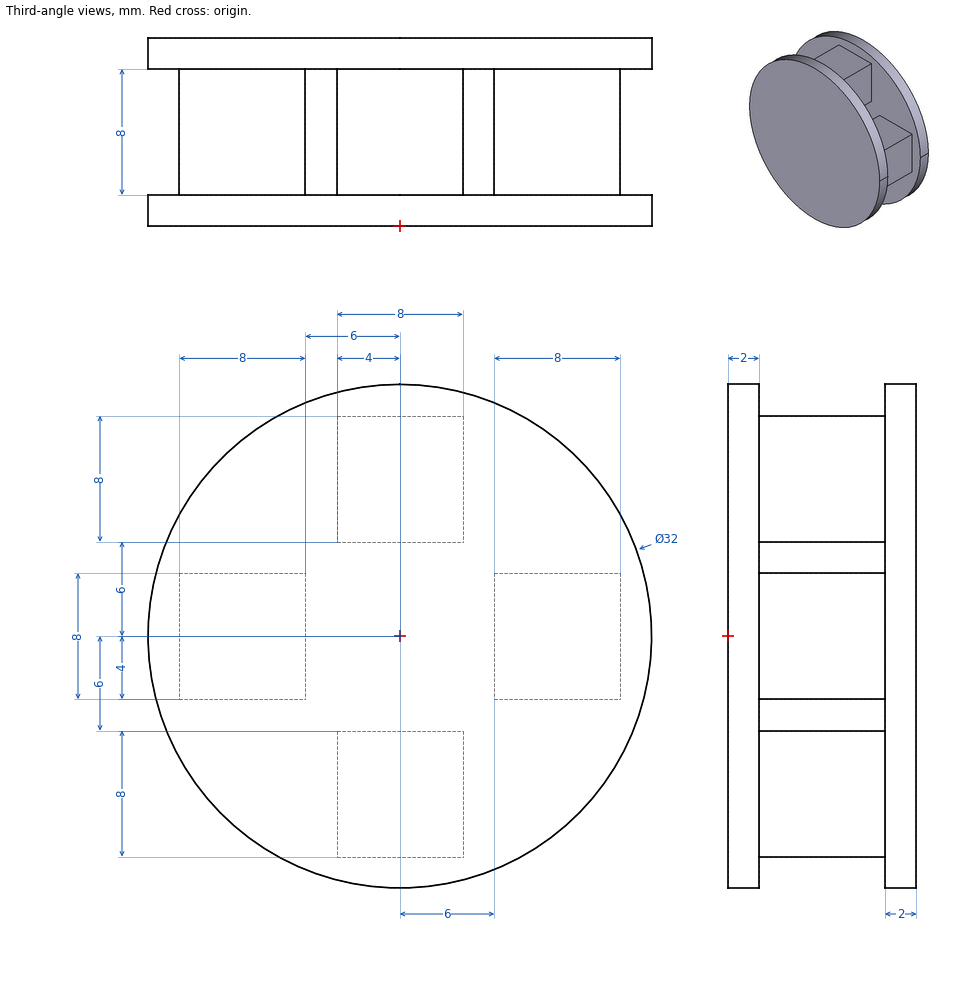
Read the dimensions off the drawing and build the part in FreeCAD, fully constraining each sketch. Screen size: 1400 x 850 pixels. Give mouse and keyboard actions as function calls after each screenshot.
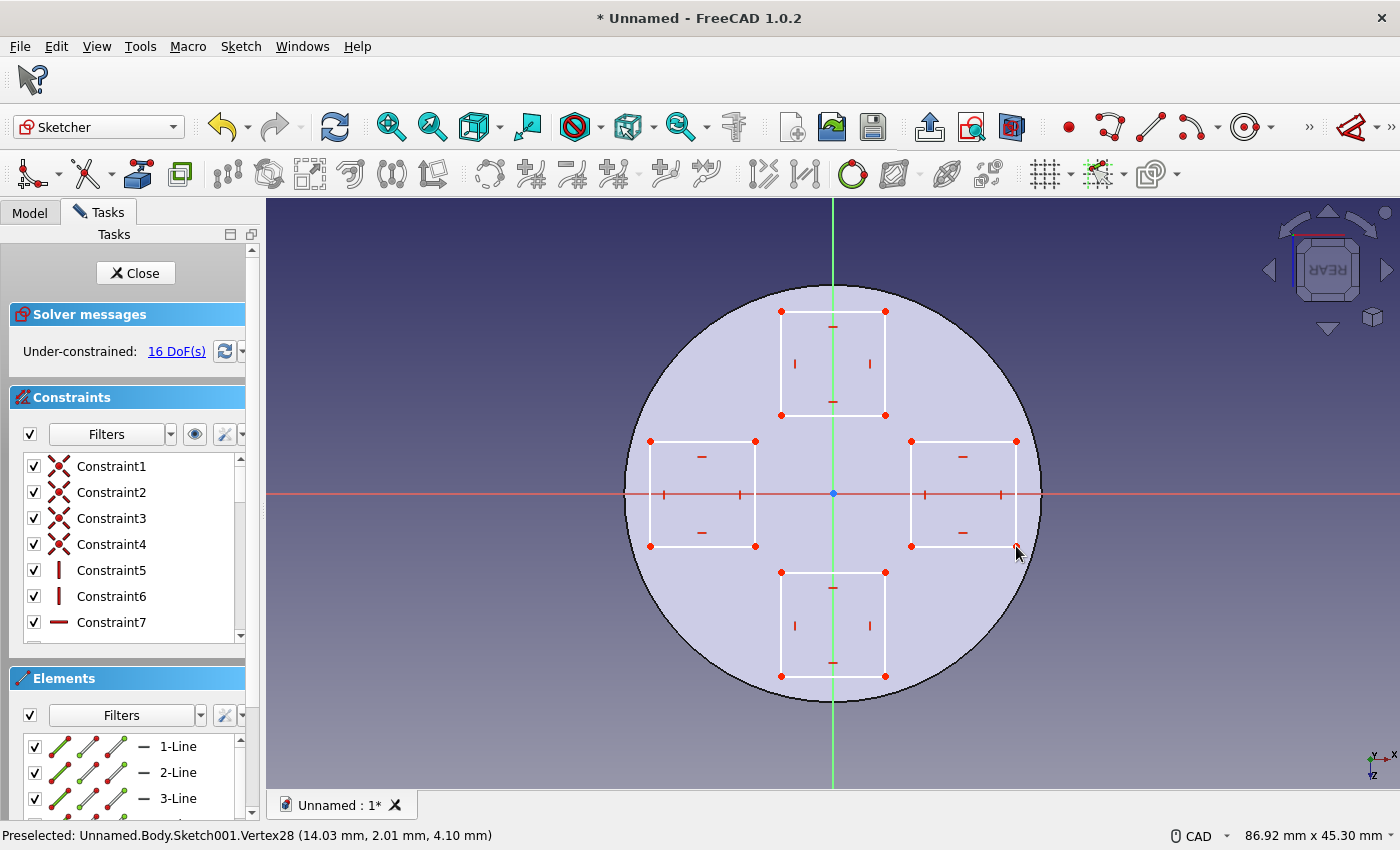
key(d)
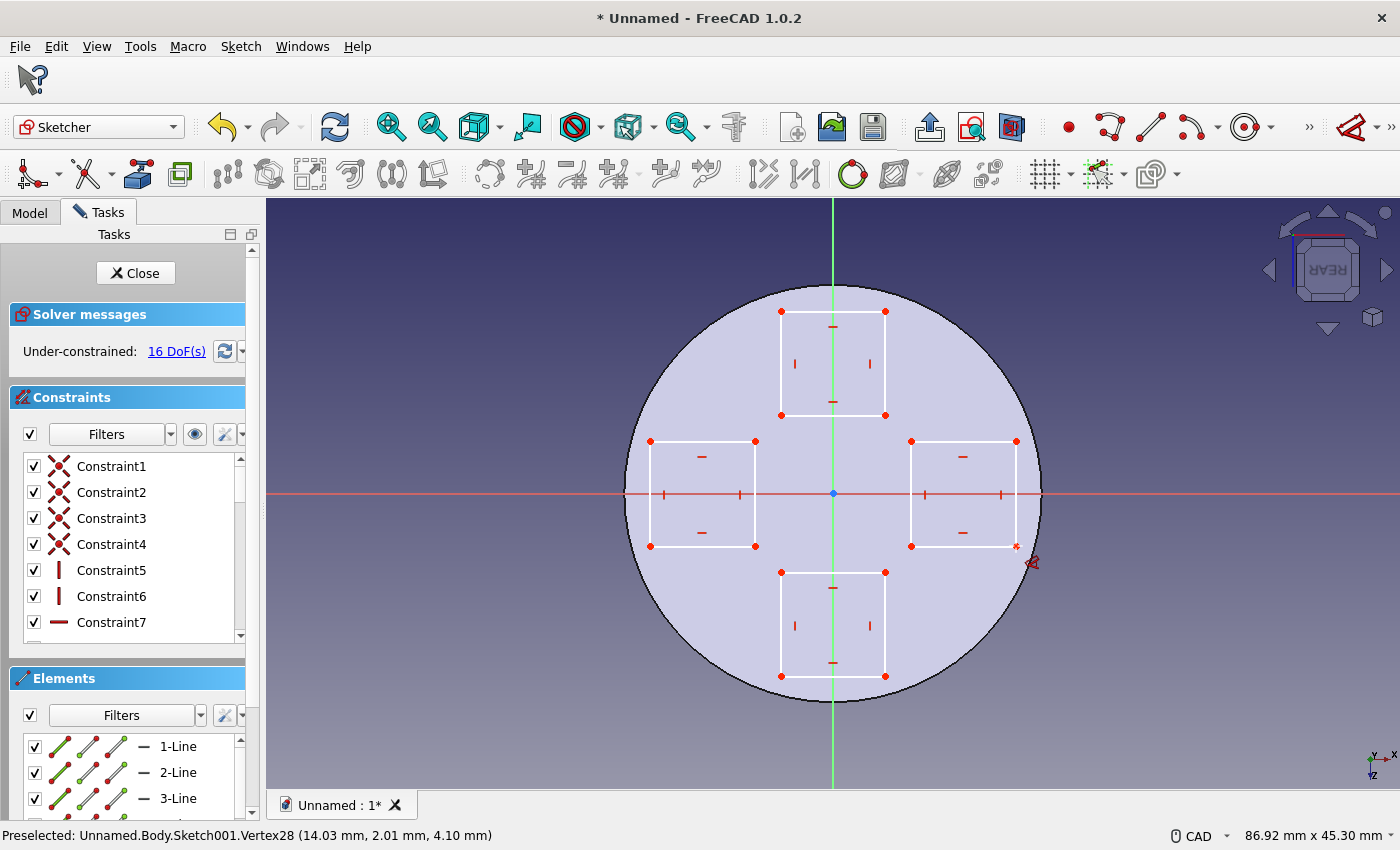
click(650, 473)
click(616, 470)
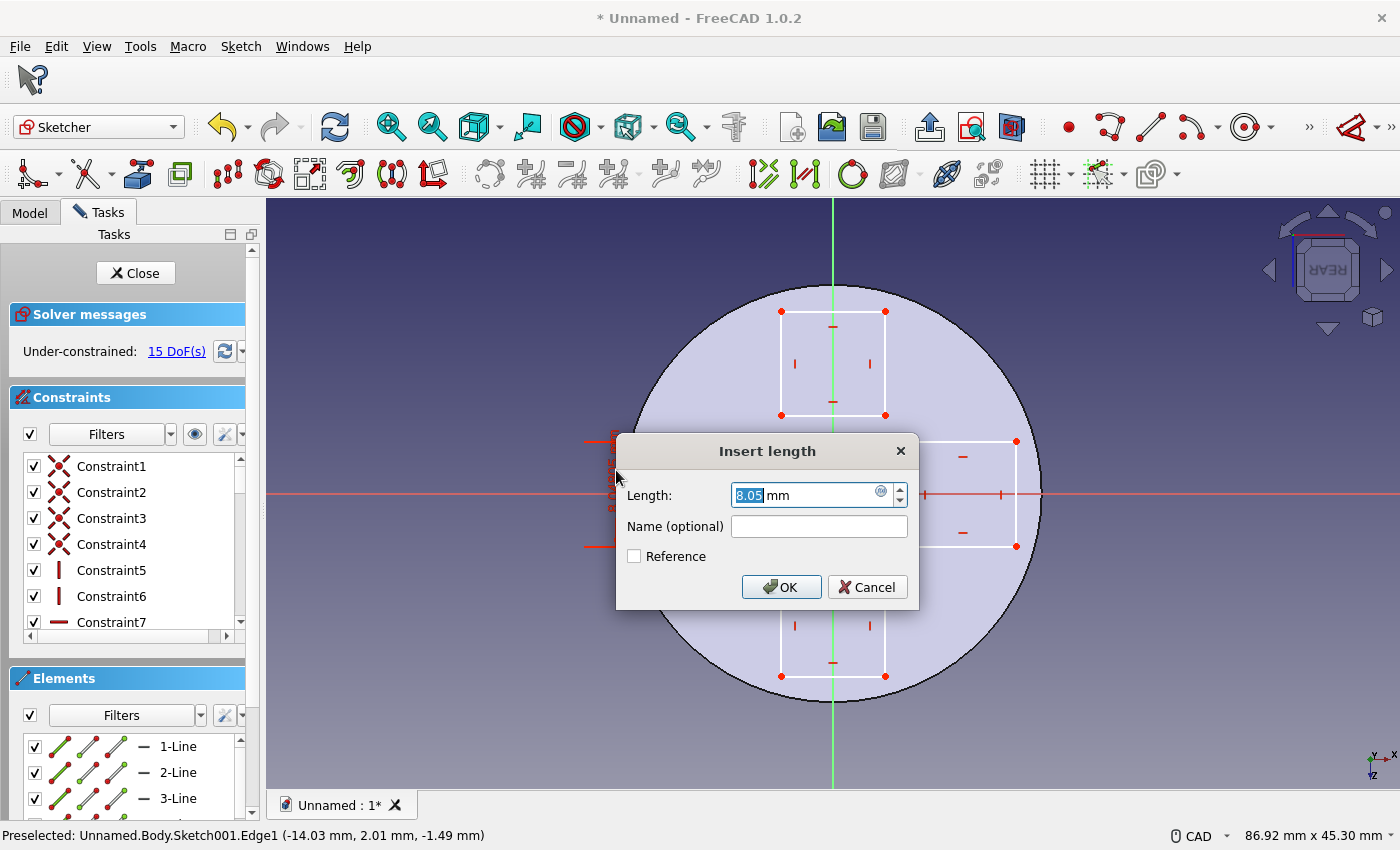
text(8)
key(Return)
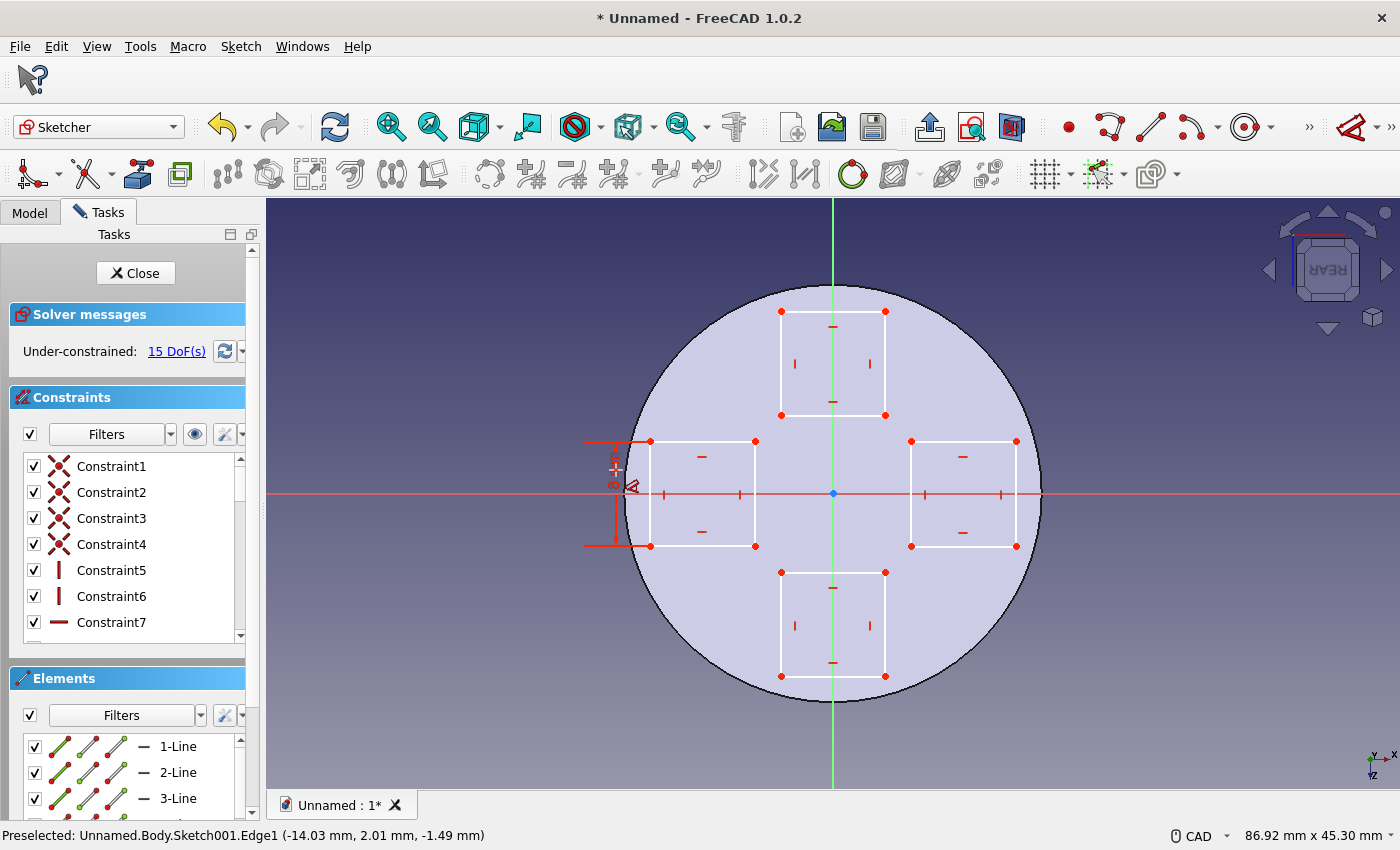
click(681, 546)
click(702, 580)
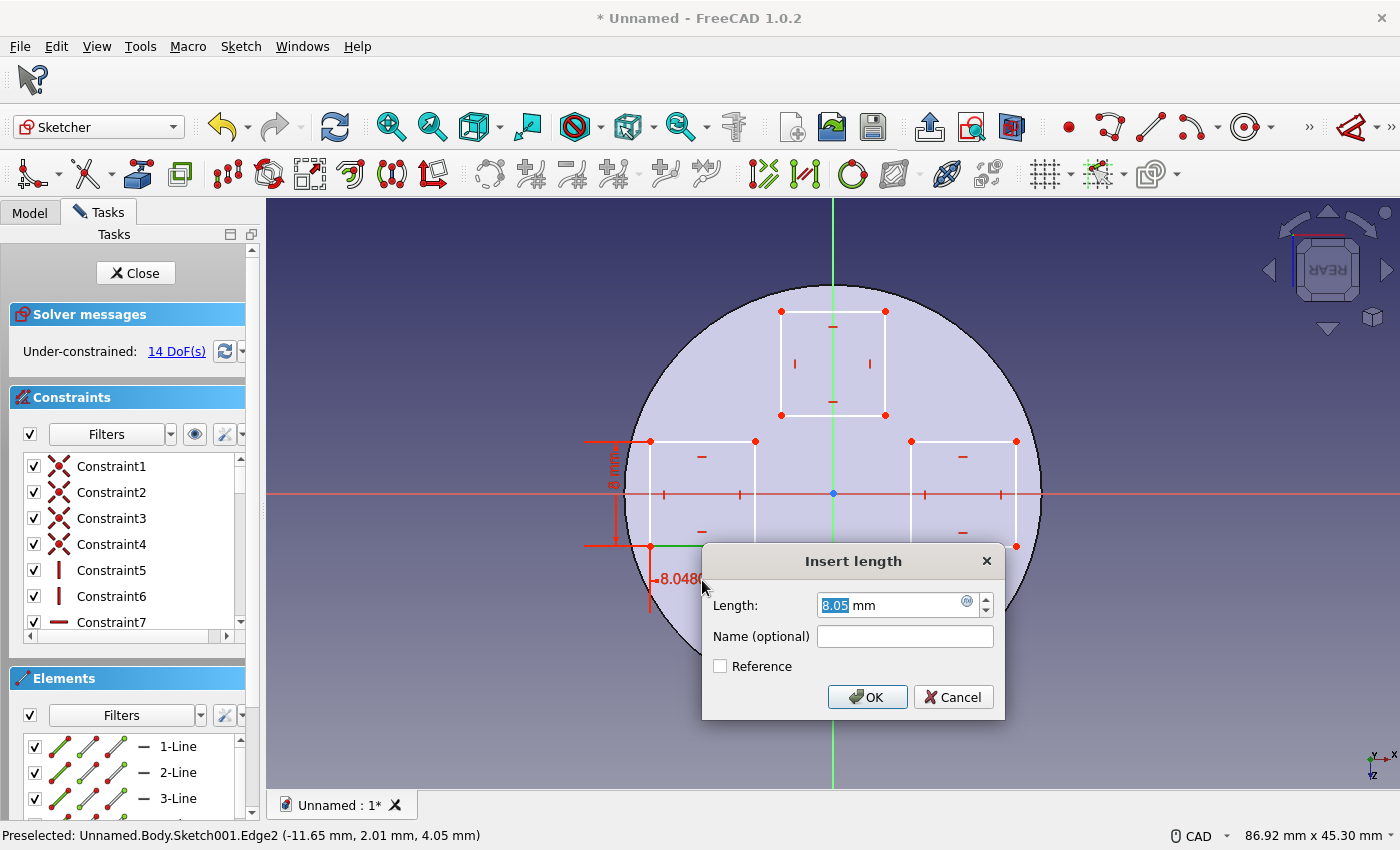
text(8)
key(Return)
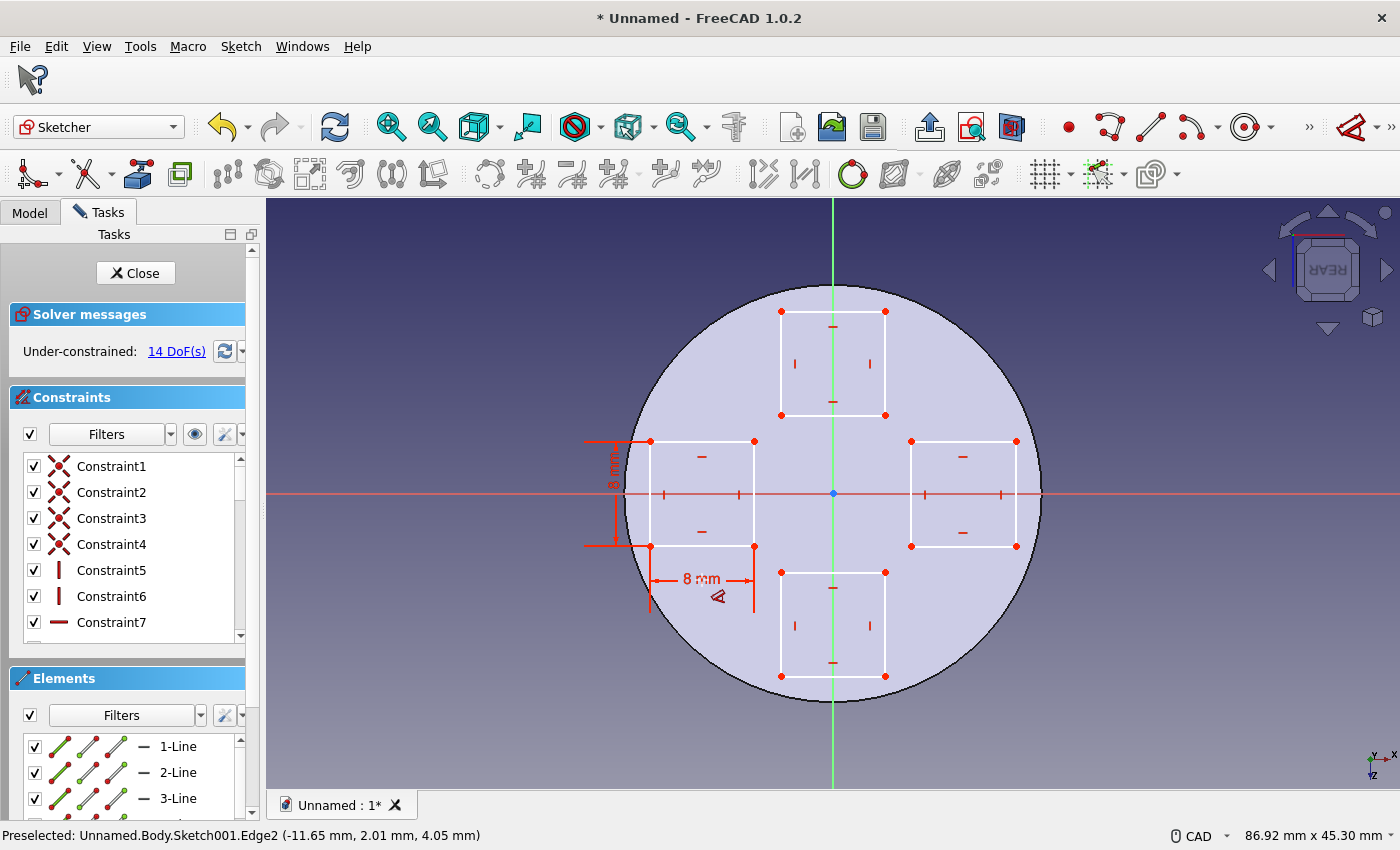
click(781, 604)
click(747, 625)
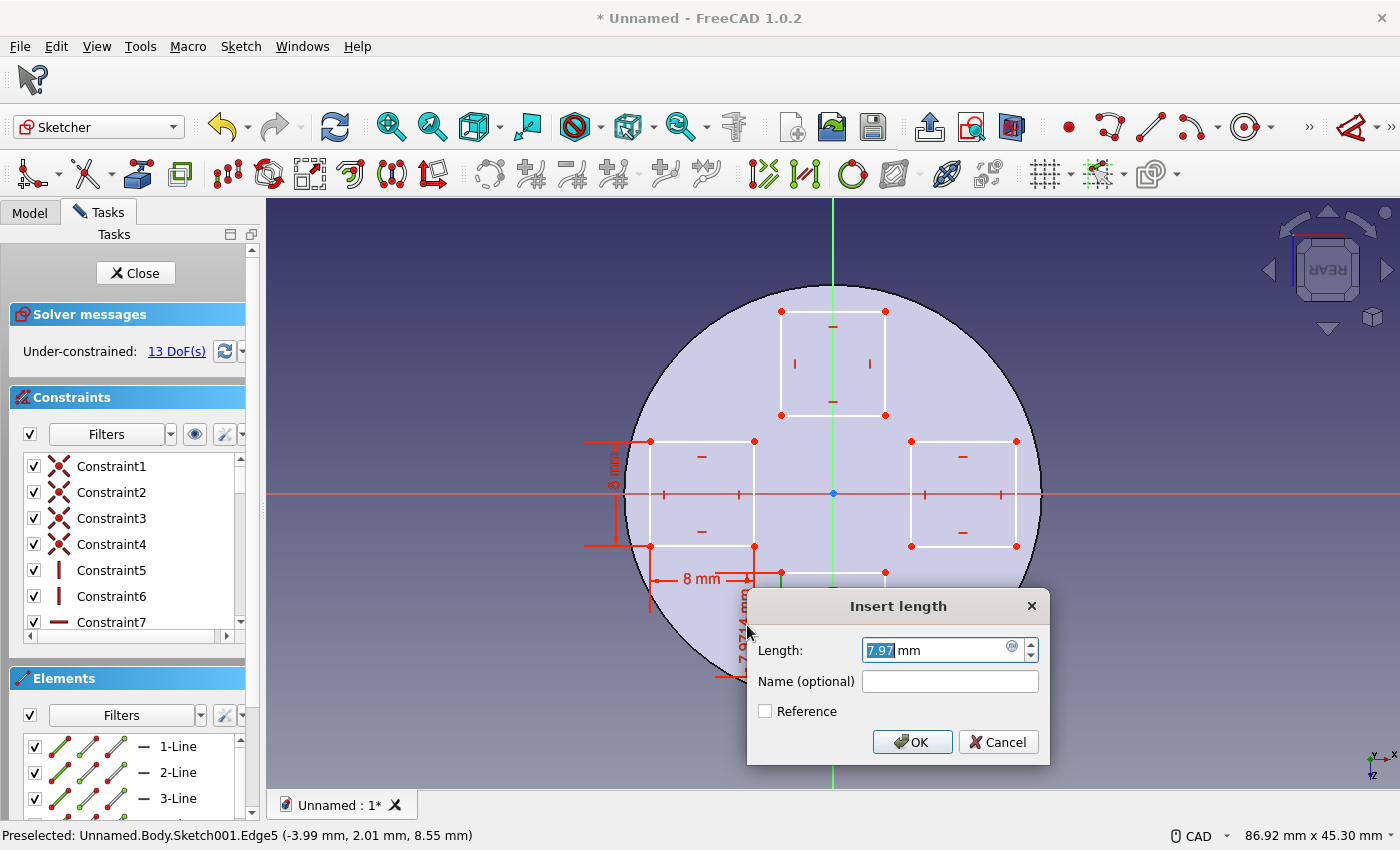
text(8)
key(Return)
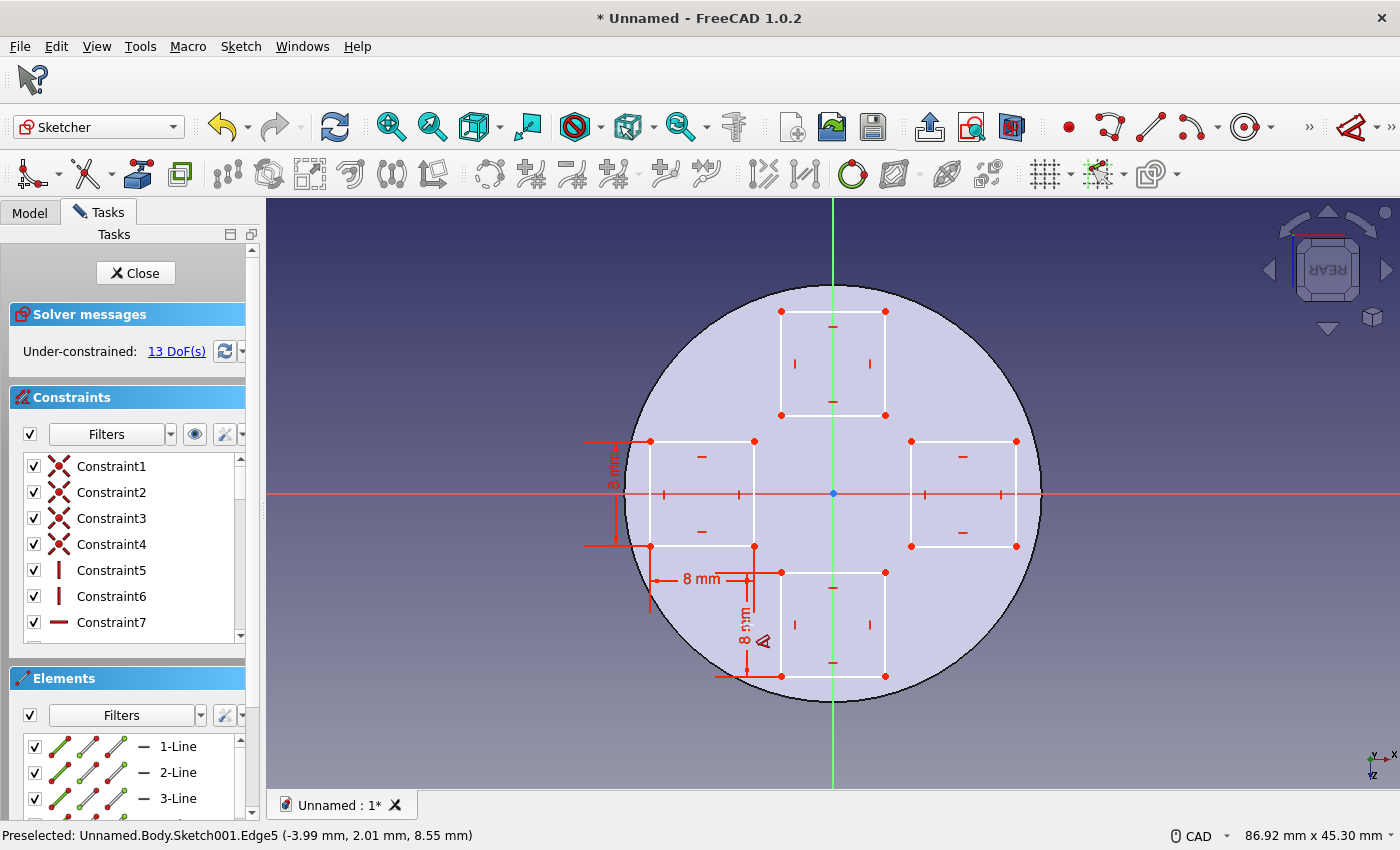
click(812, 677)
click(809, 711)